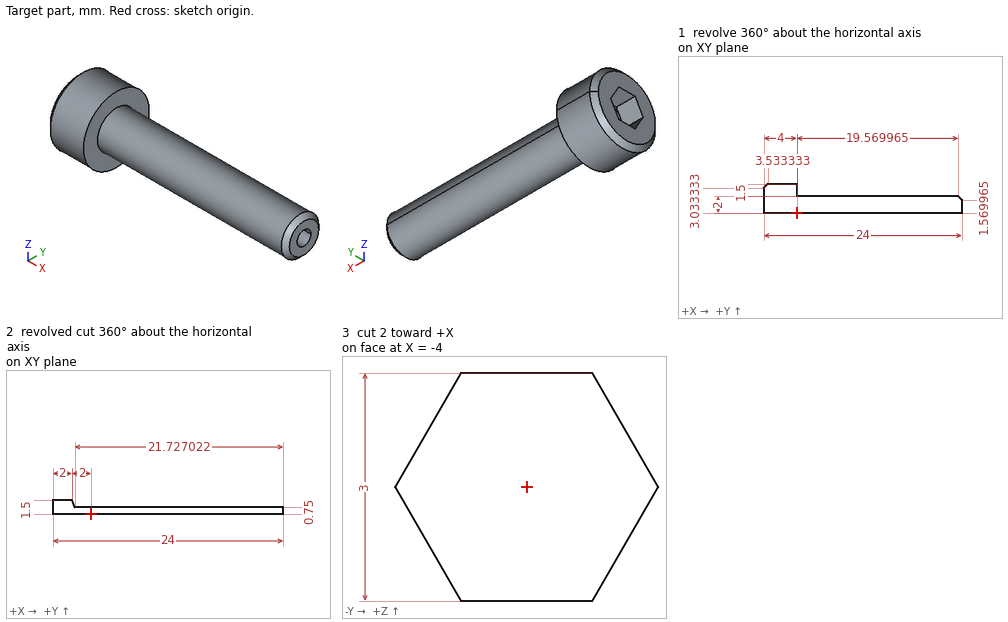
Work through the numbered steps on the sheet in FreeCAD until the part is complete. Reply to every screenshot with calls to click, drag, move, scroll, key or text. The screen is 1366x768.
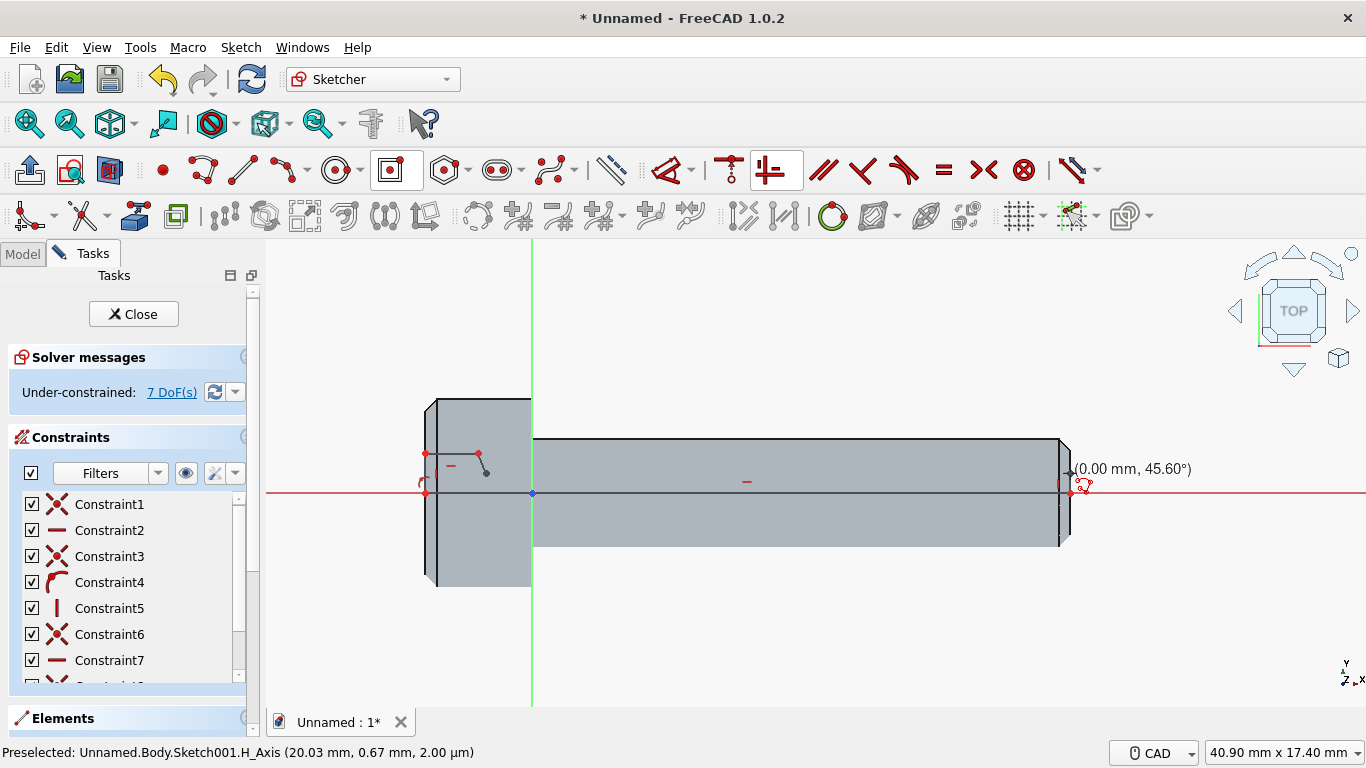
scroll(486, 473, up, 2)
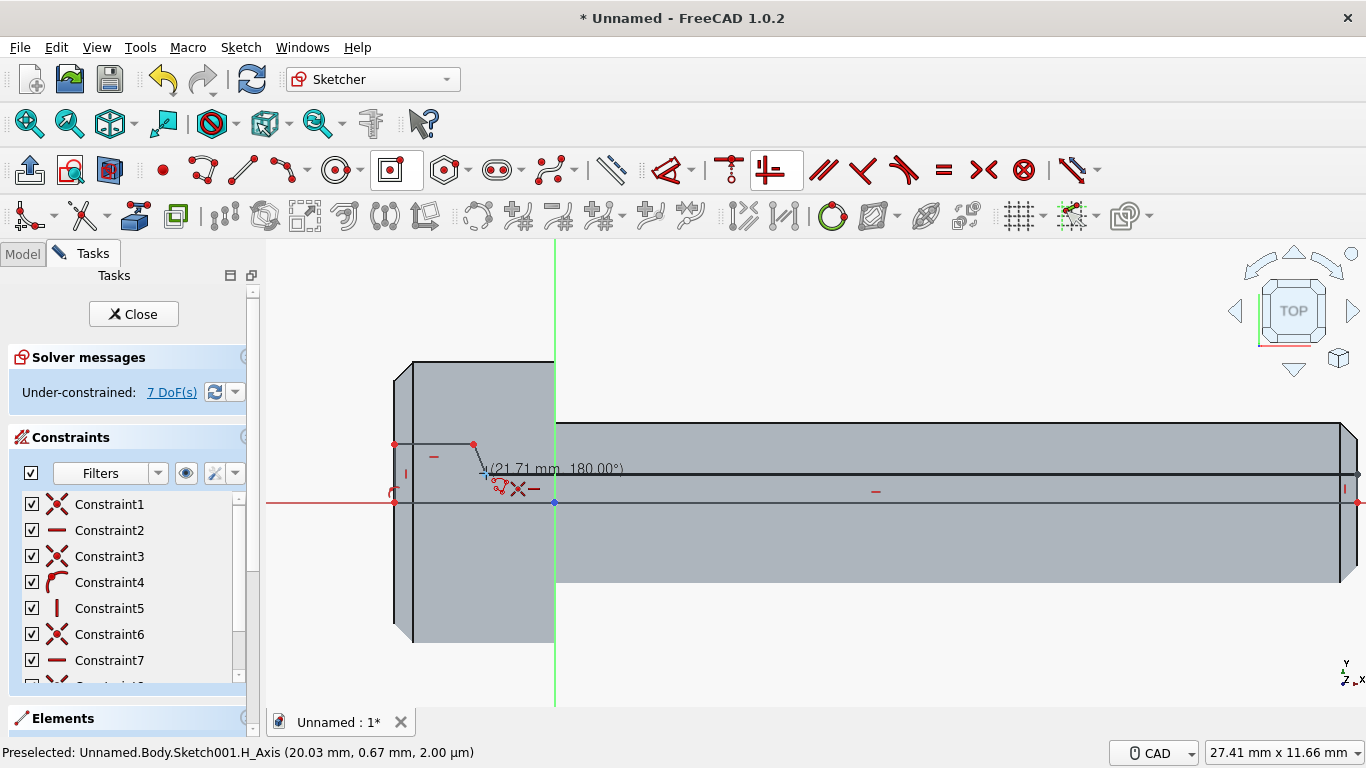
click(486, 474)
key(Escape)
key(Escape)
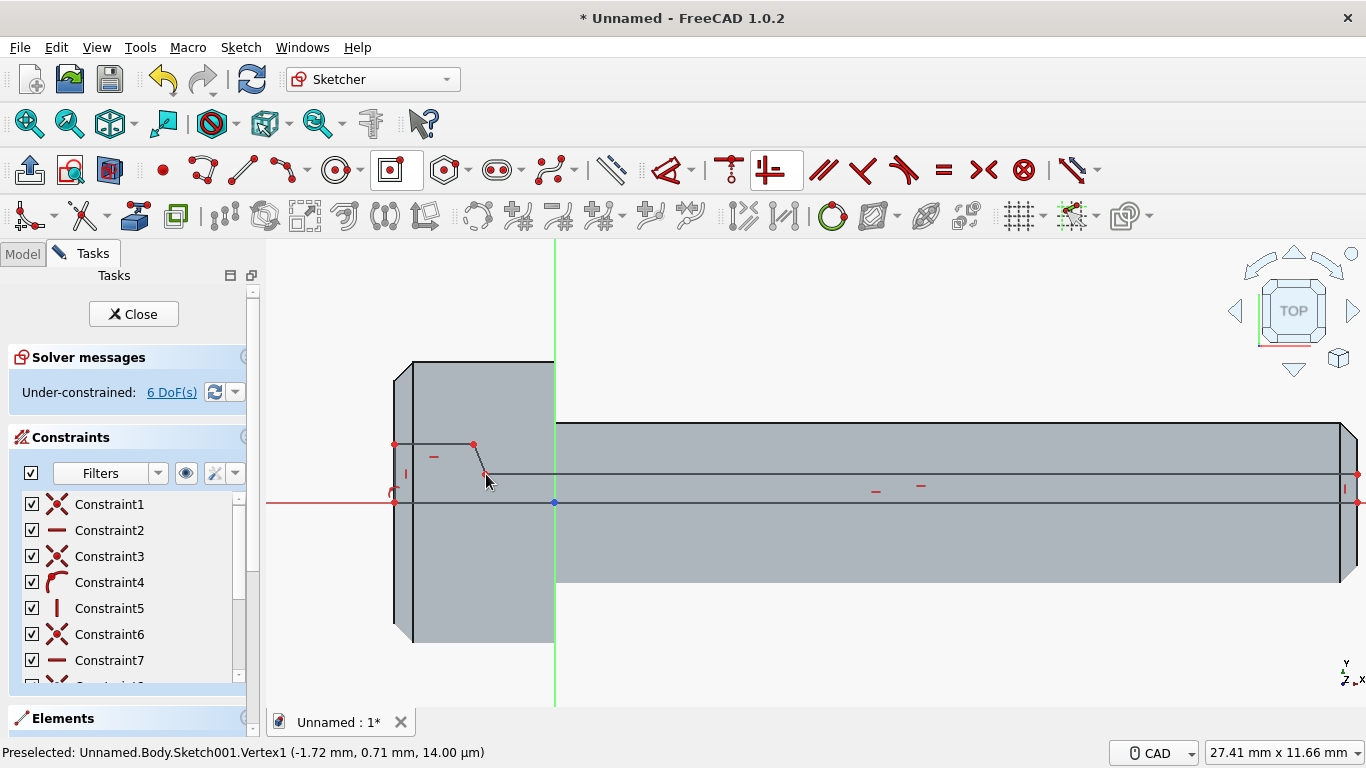
click(666, 170)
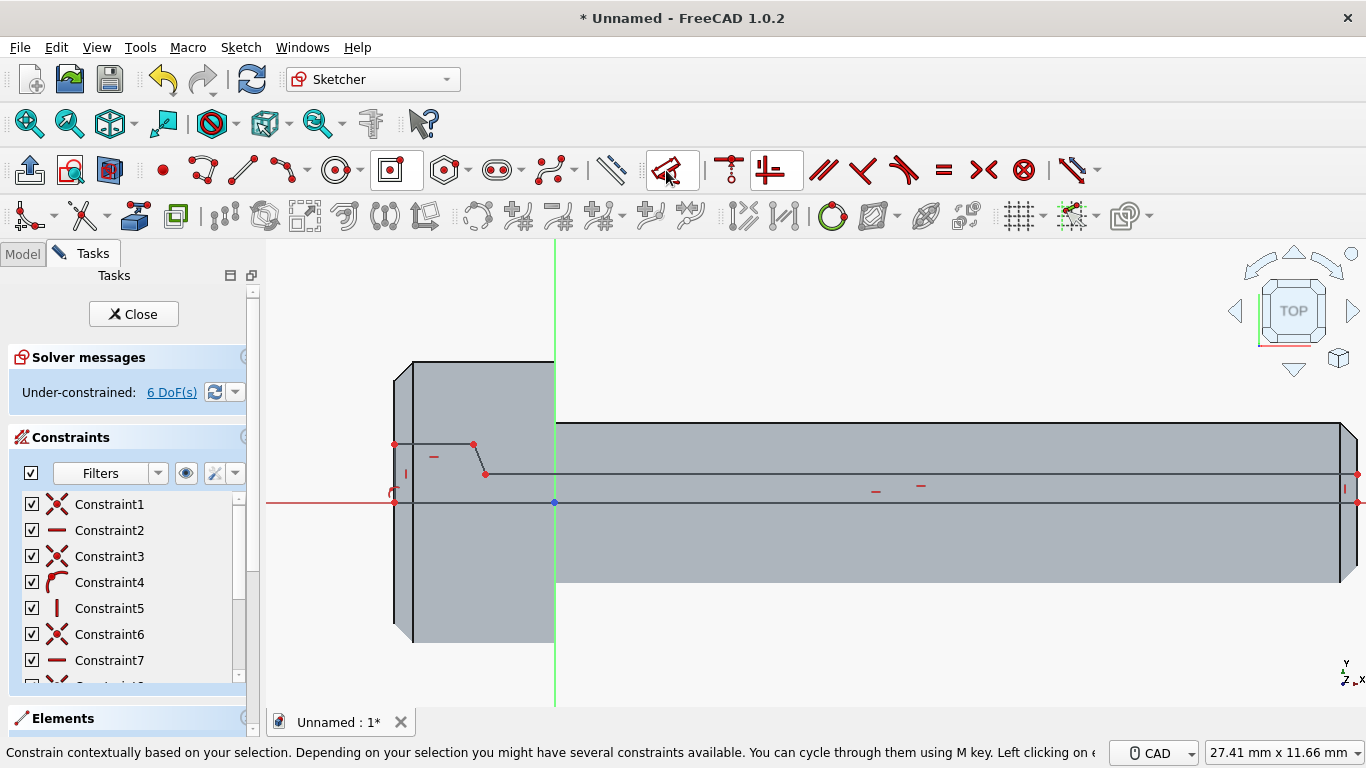
click(450, 444)
click(434, 410)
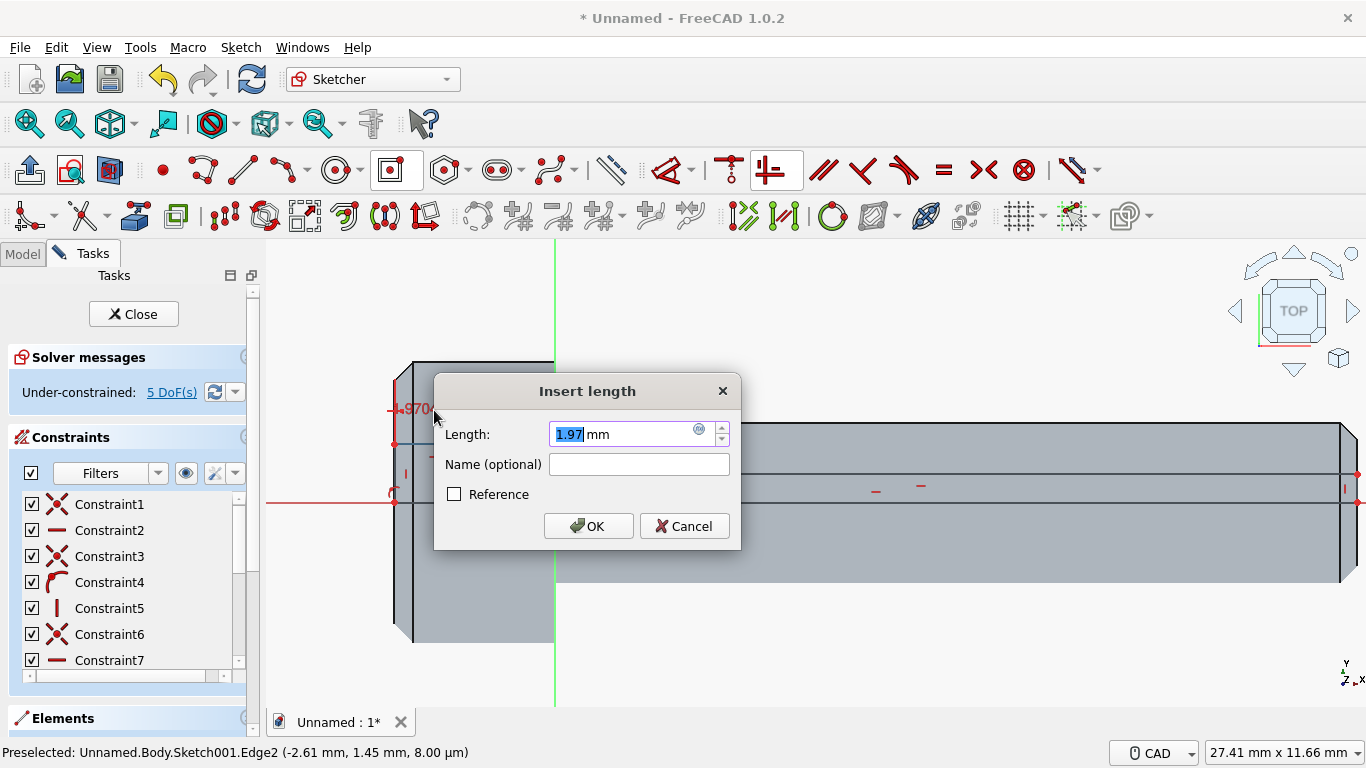
text(2)
key(Return)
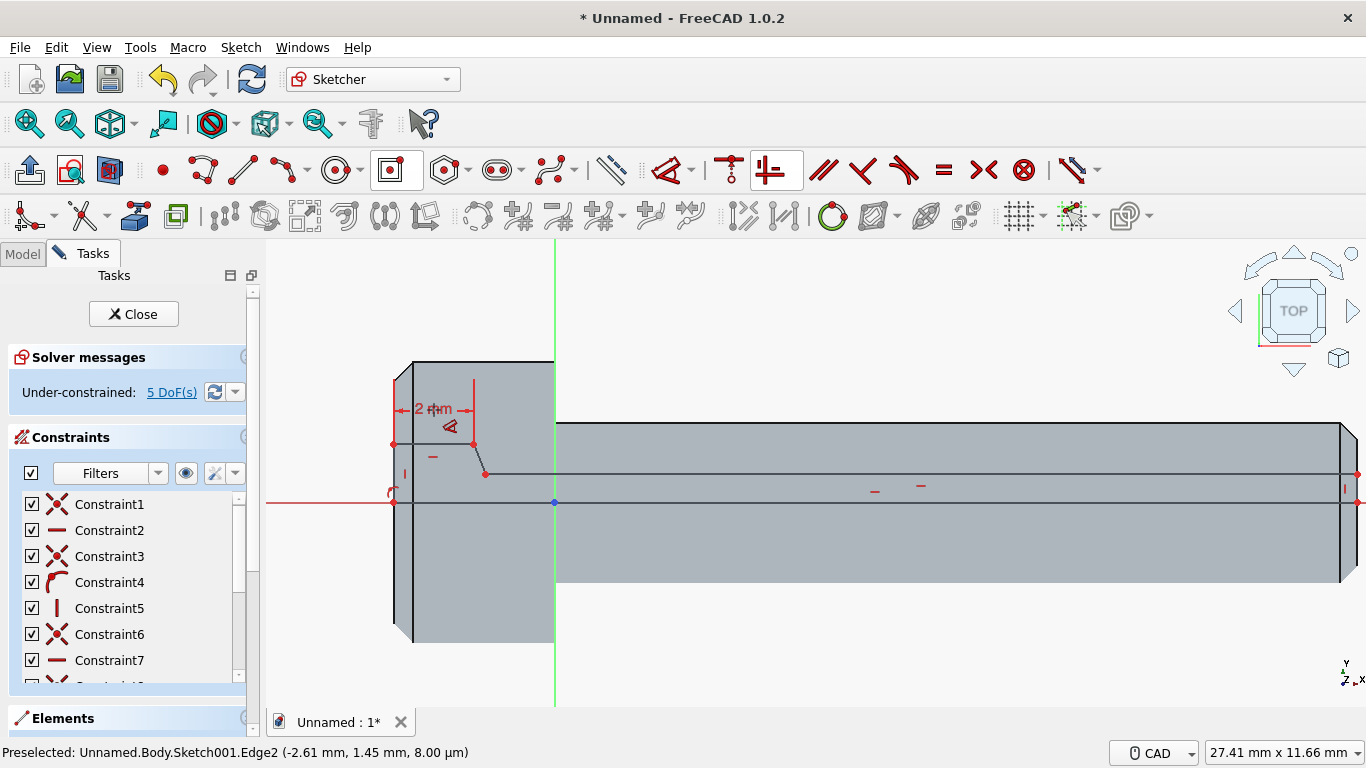
click(683, 503)
click(797, 537)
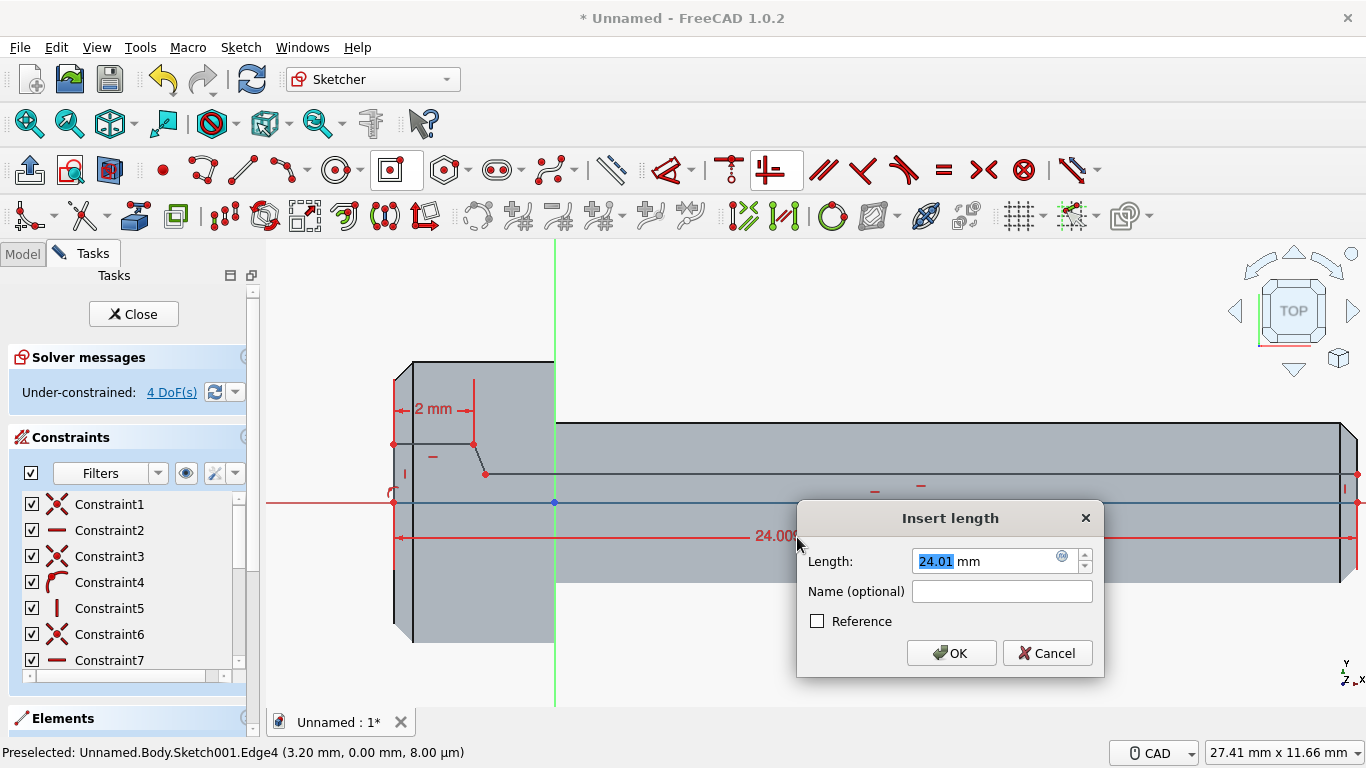
text(24)
key(Return)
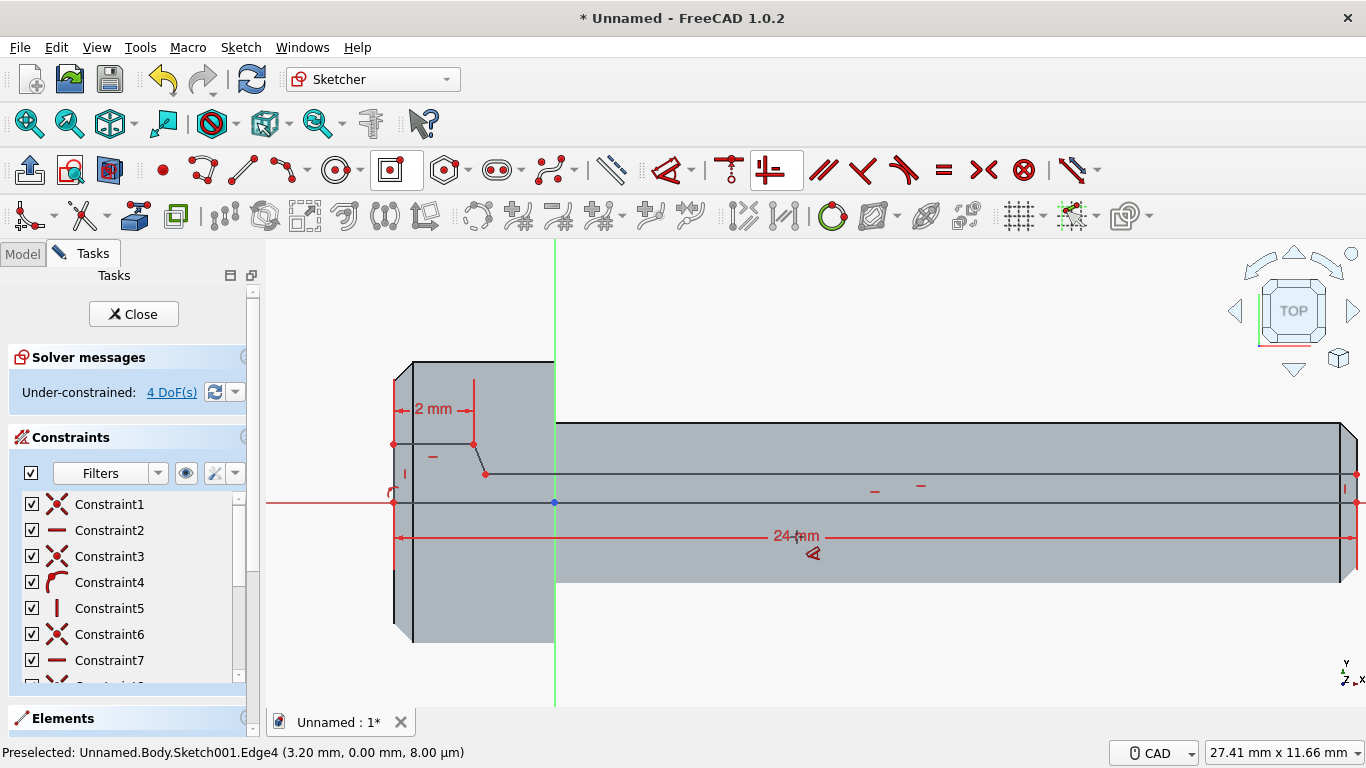
click(474, 444)
click(514, 537)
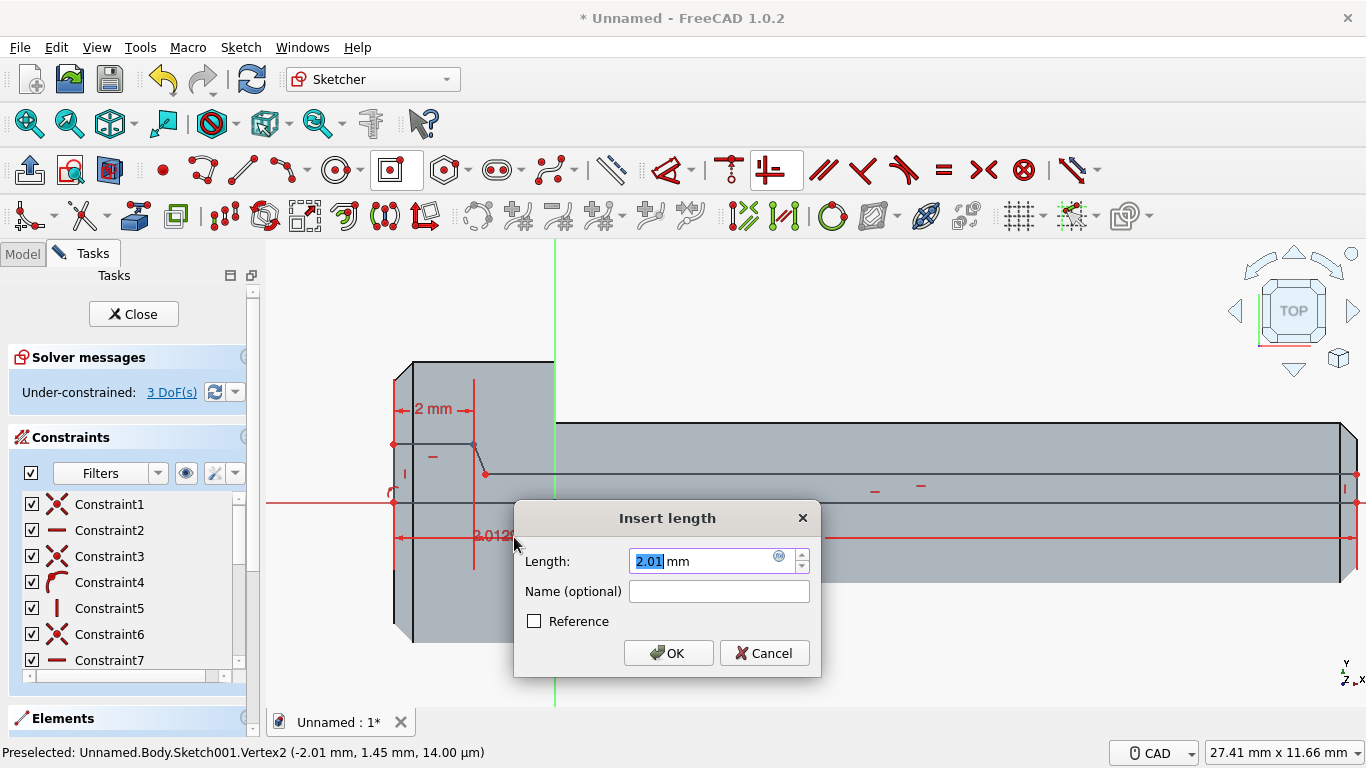
text(2)
key(Return)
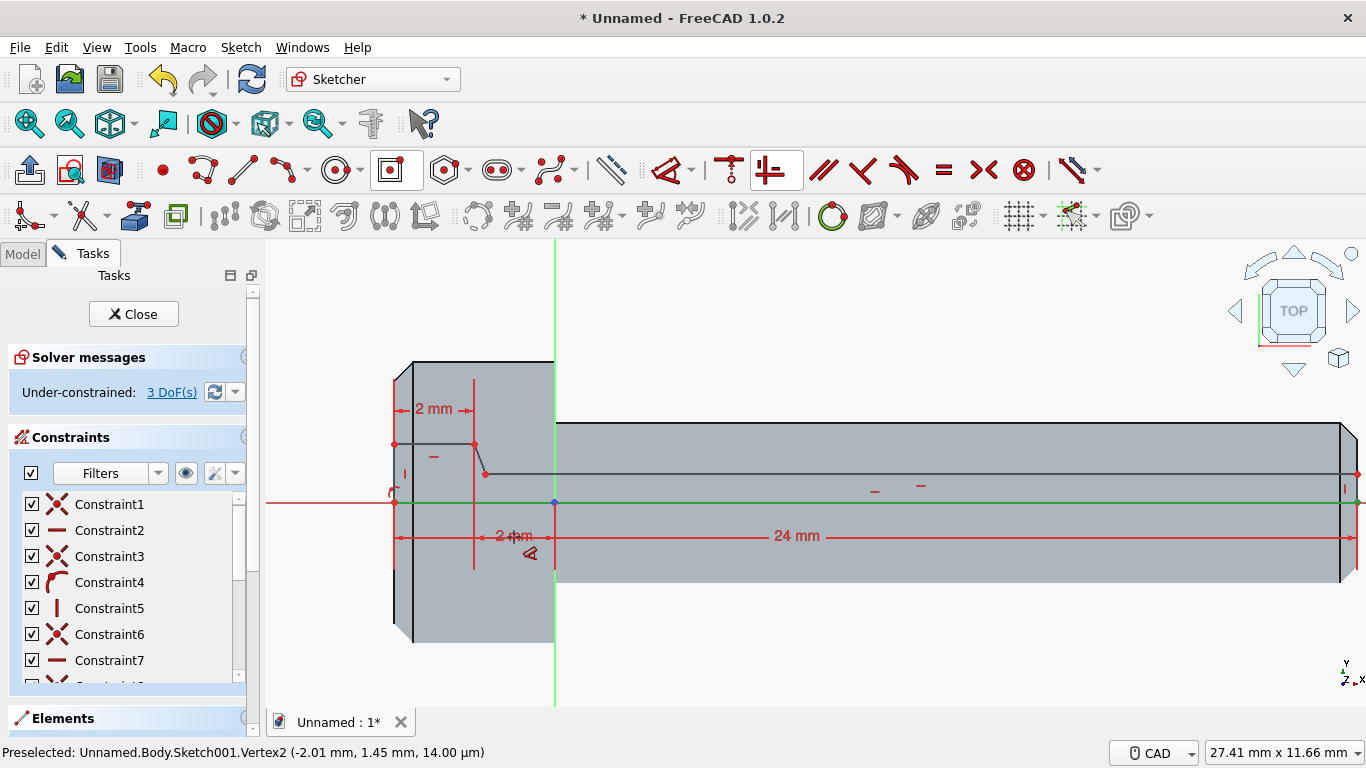
click(394, 462)
click(360, 474)